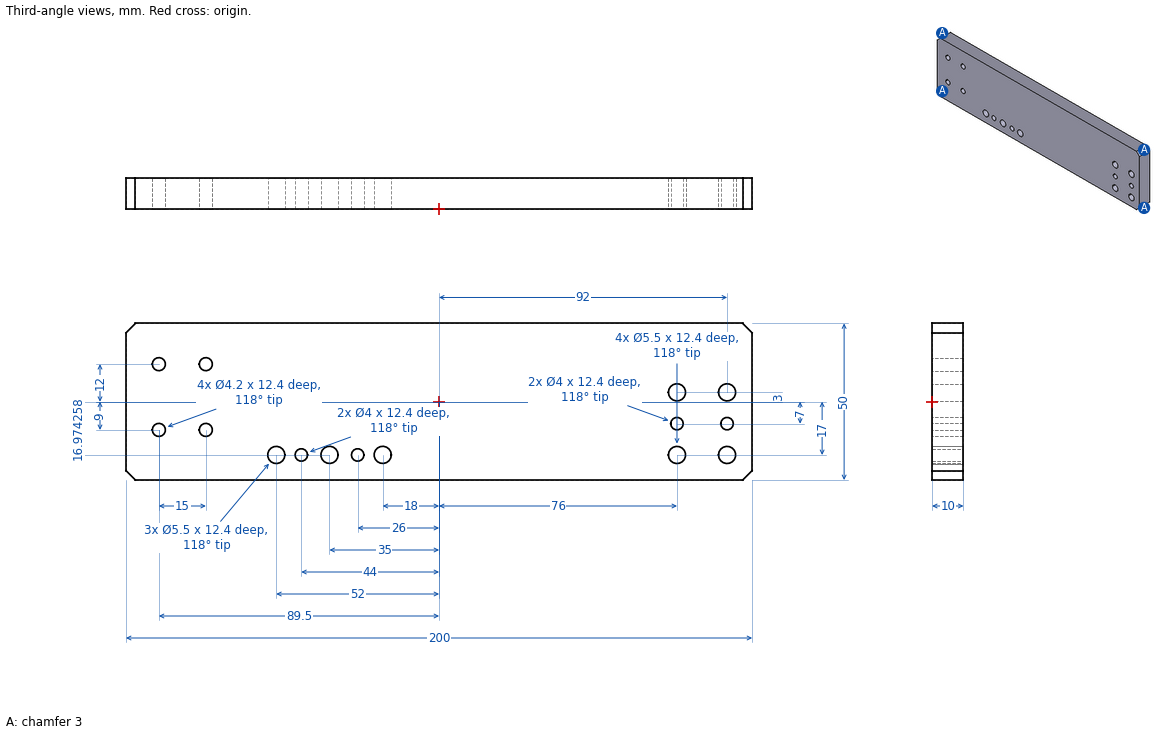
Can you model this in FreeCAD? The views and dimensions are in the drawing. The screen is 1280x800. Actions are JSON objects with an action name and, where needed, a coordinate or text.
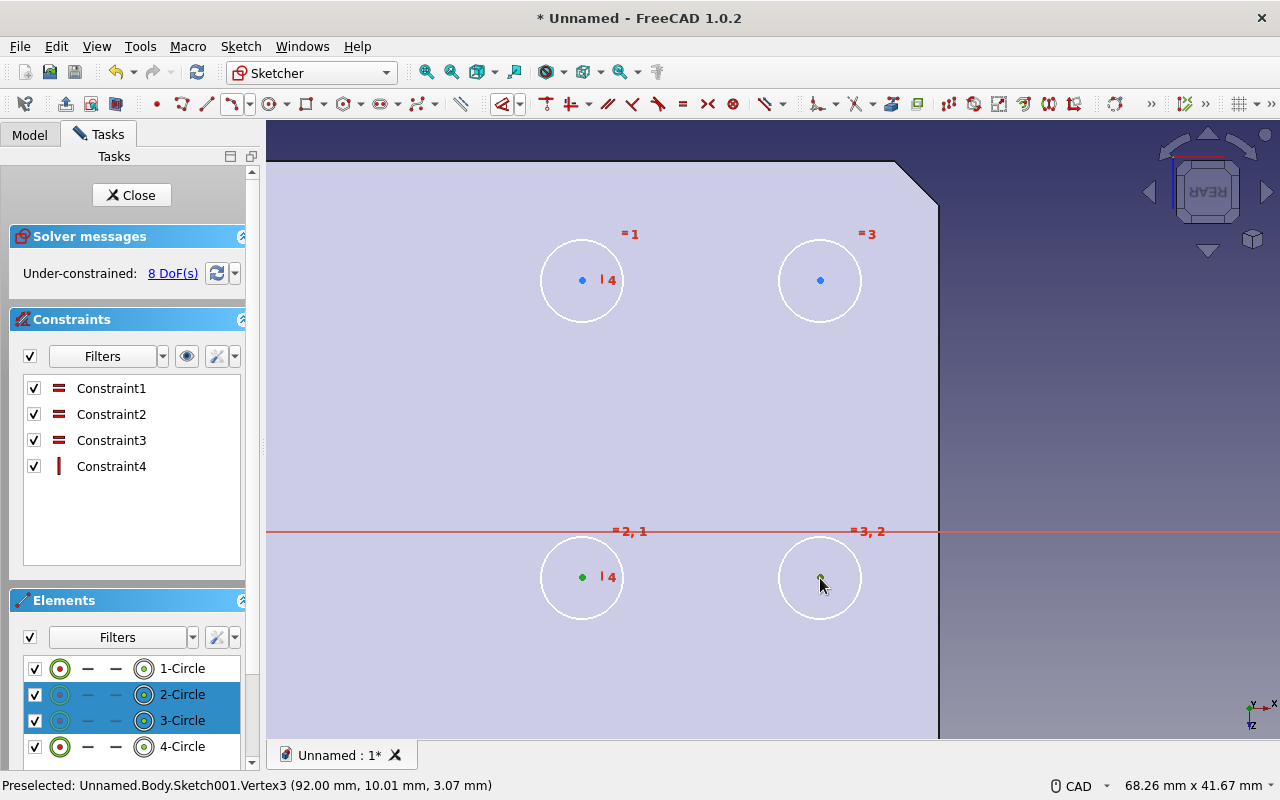
{"action": "key", "text": "h"}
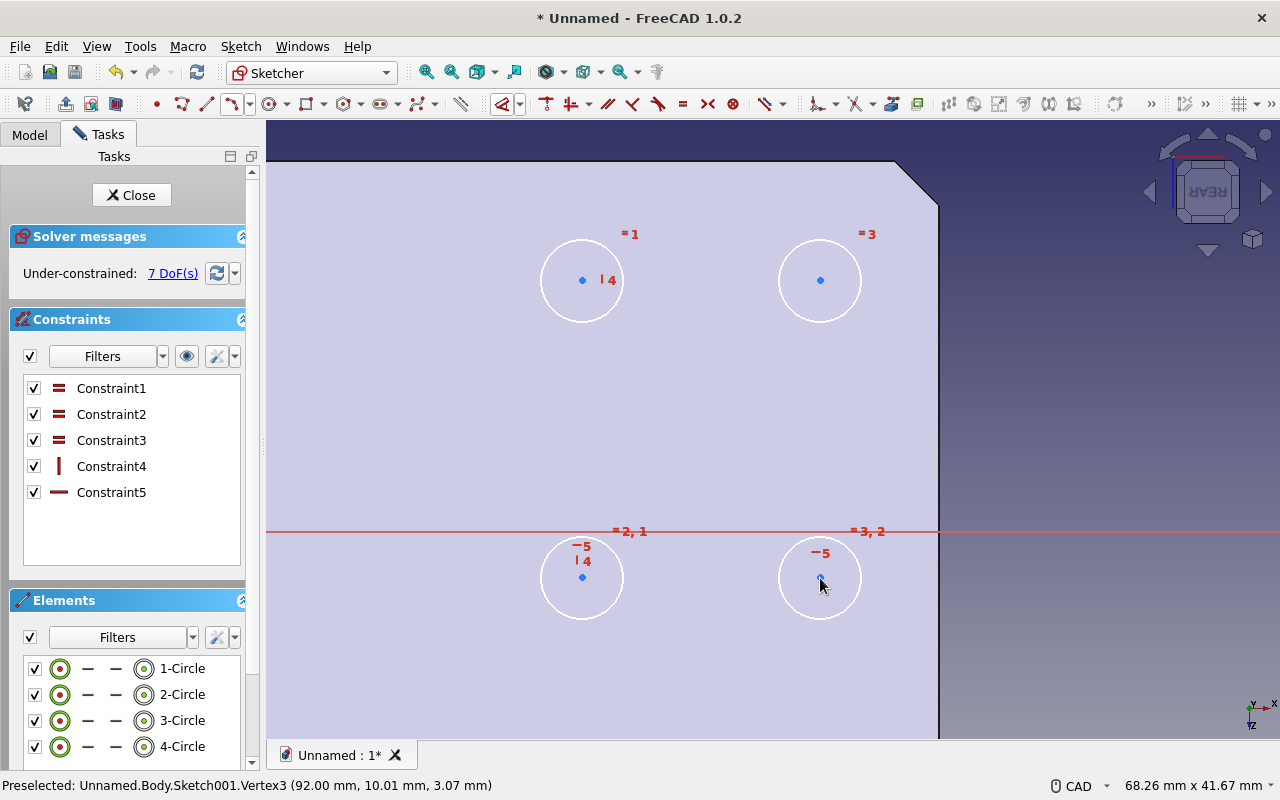
{"action": "left_click", "coordinate": [820, 578]}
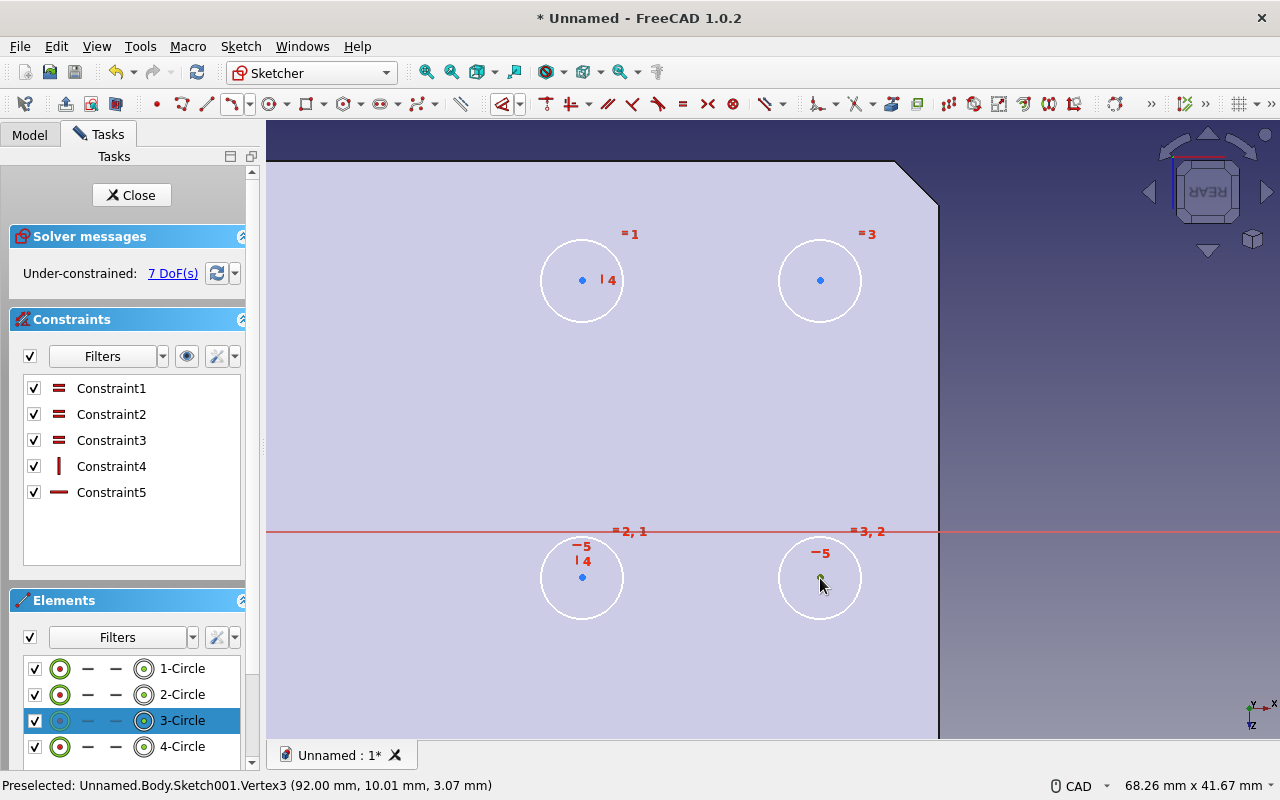
{"action": "left_click", "coordinate": [820, 281]}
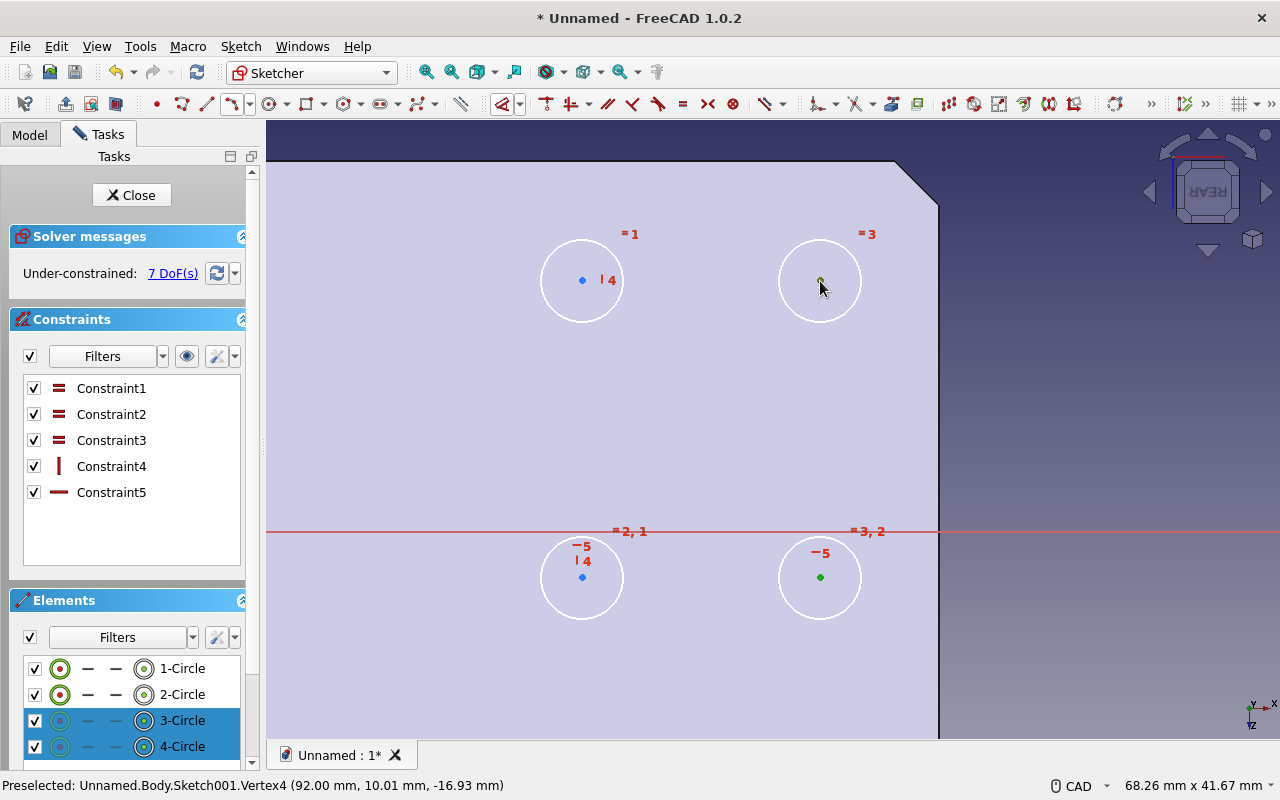
{"action": "key", "text": "v"}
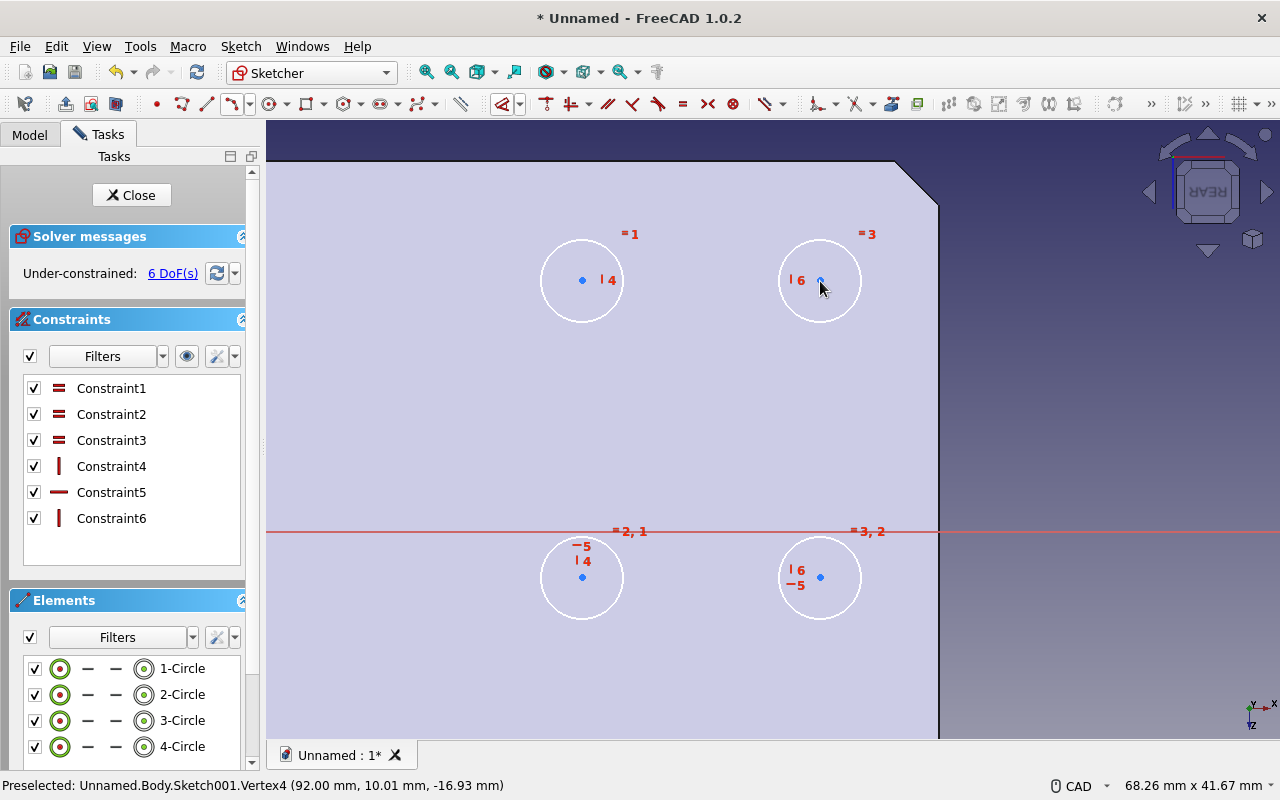
{"action": "left_click", "coordinate": [582, 281]}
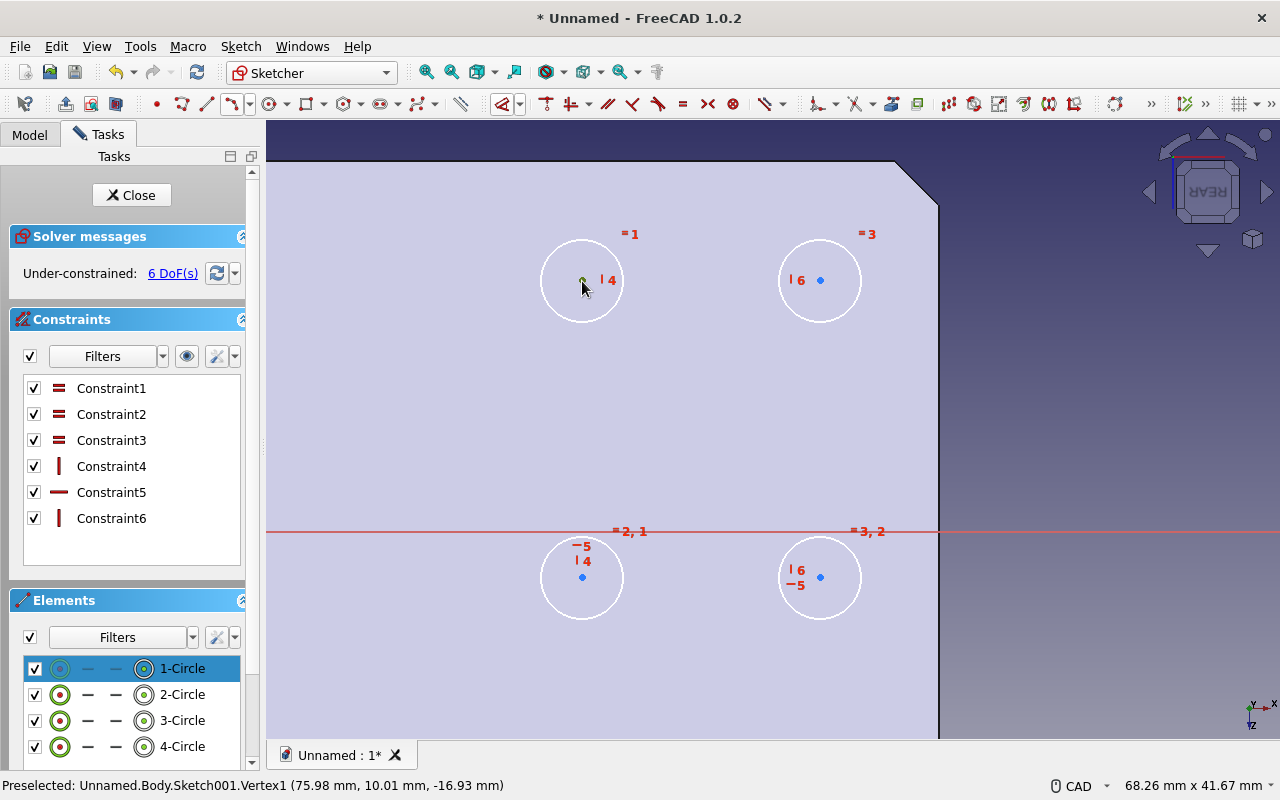
{"action": "left_click", "coordinate": [820, 281]}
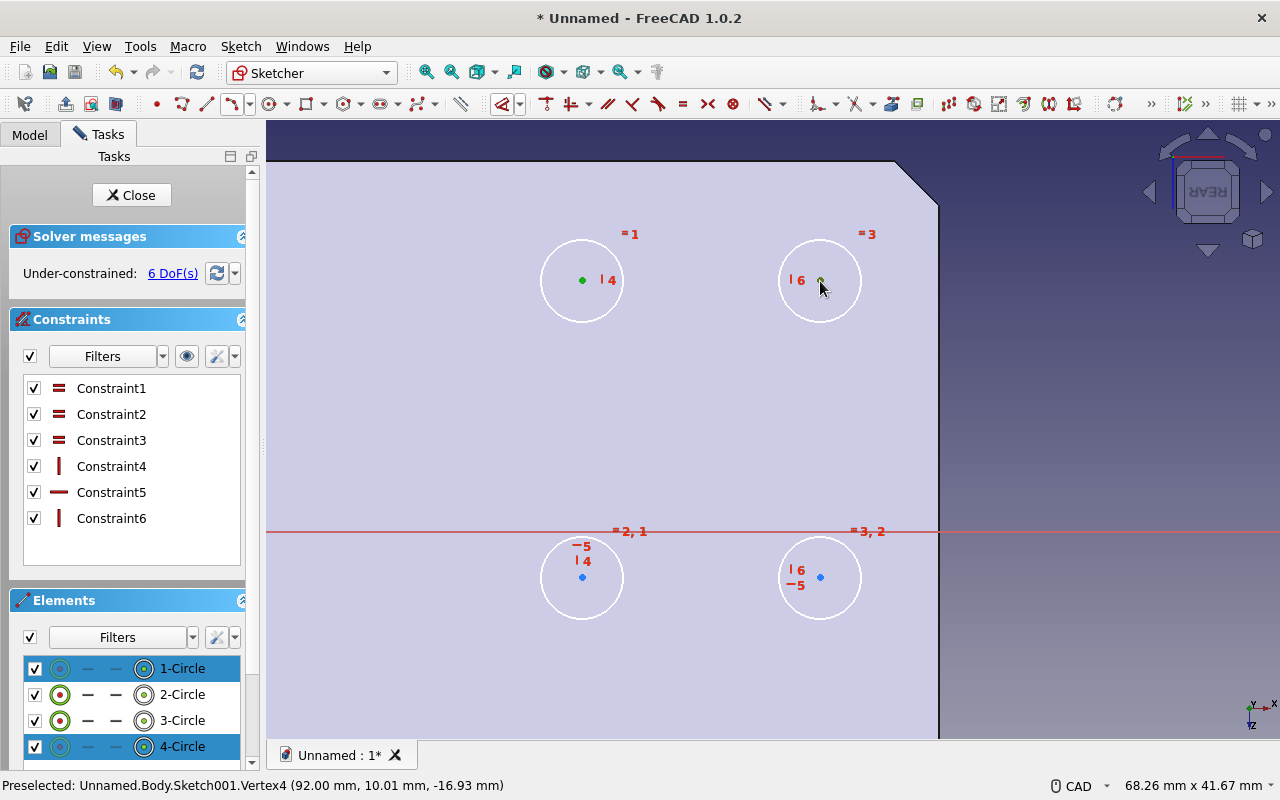
{"action": "key", "text": "h"}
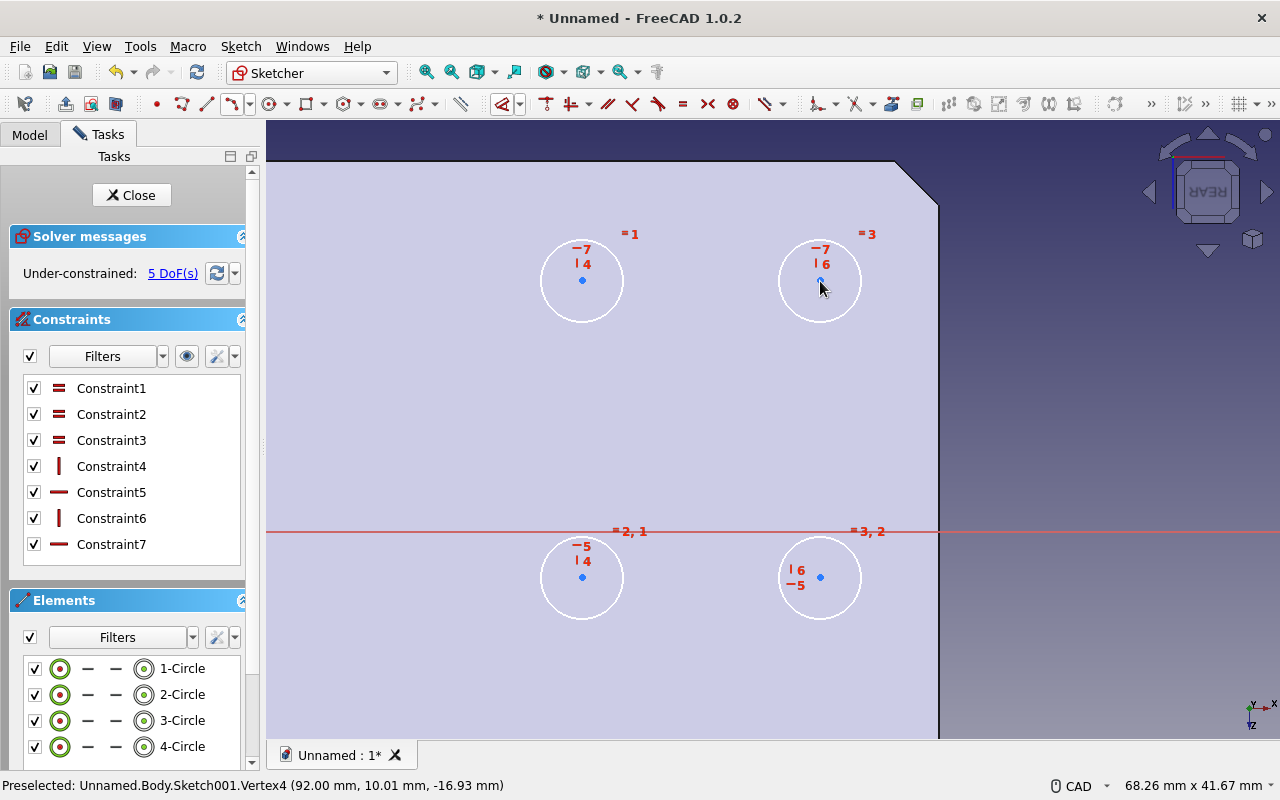
{"action": "key", "text": "d"}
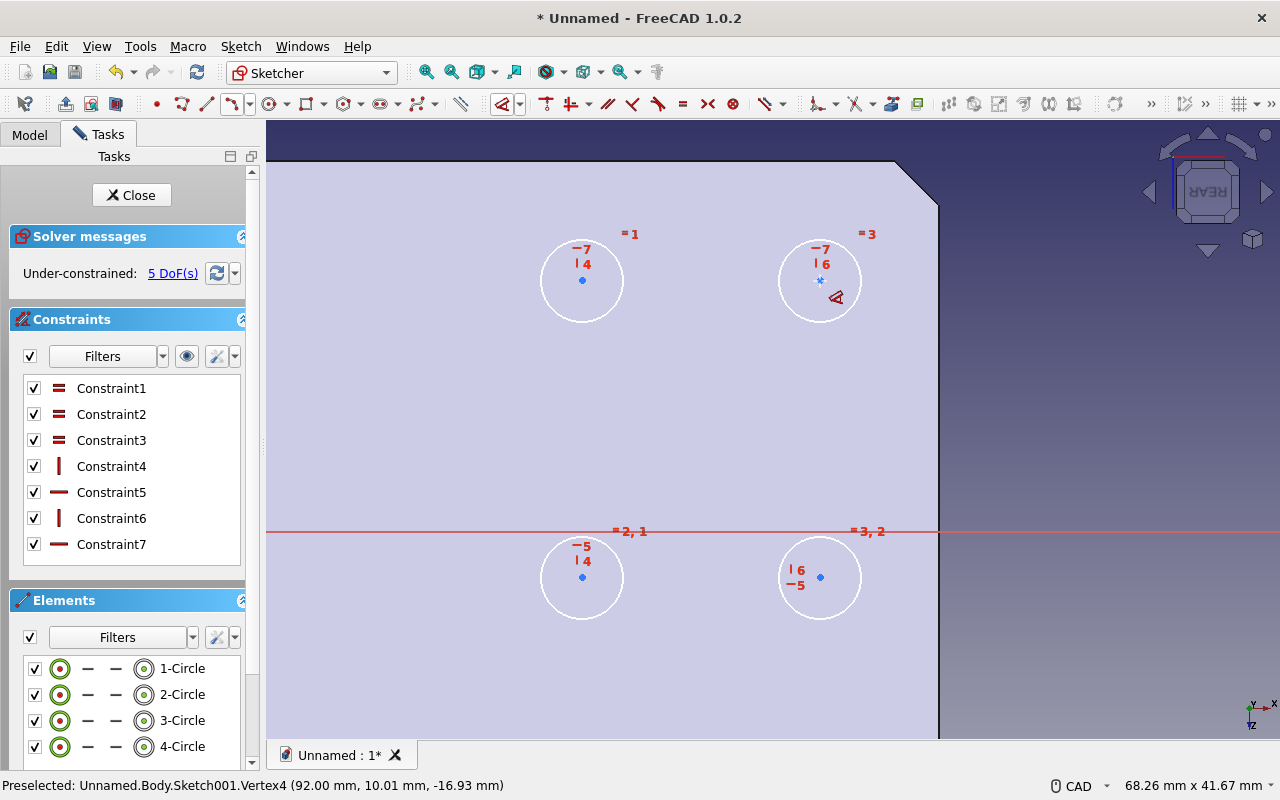
{"action": "left_click", "coordinate": [611, 252]}
{"action": "left_click", "coordinate": [634, 229]}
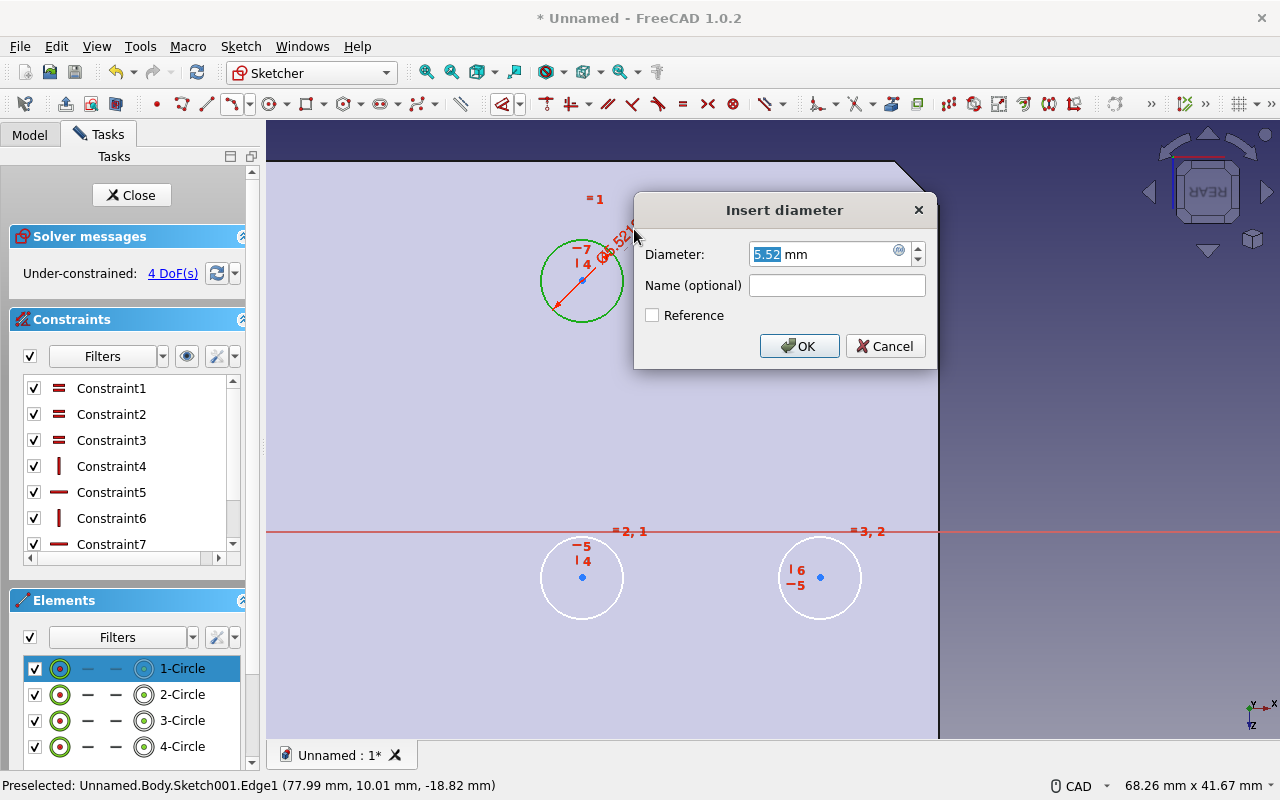
{"action": "type", "text": "5.5"}
{"action": "key", "text": "Return"}